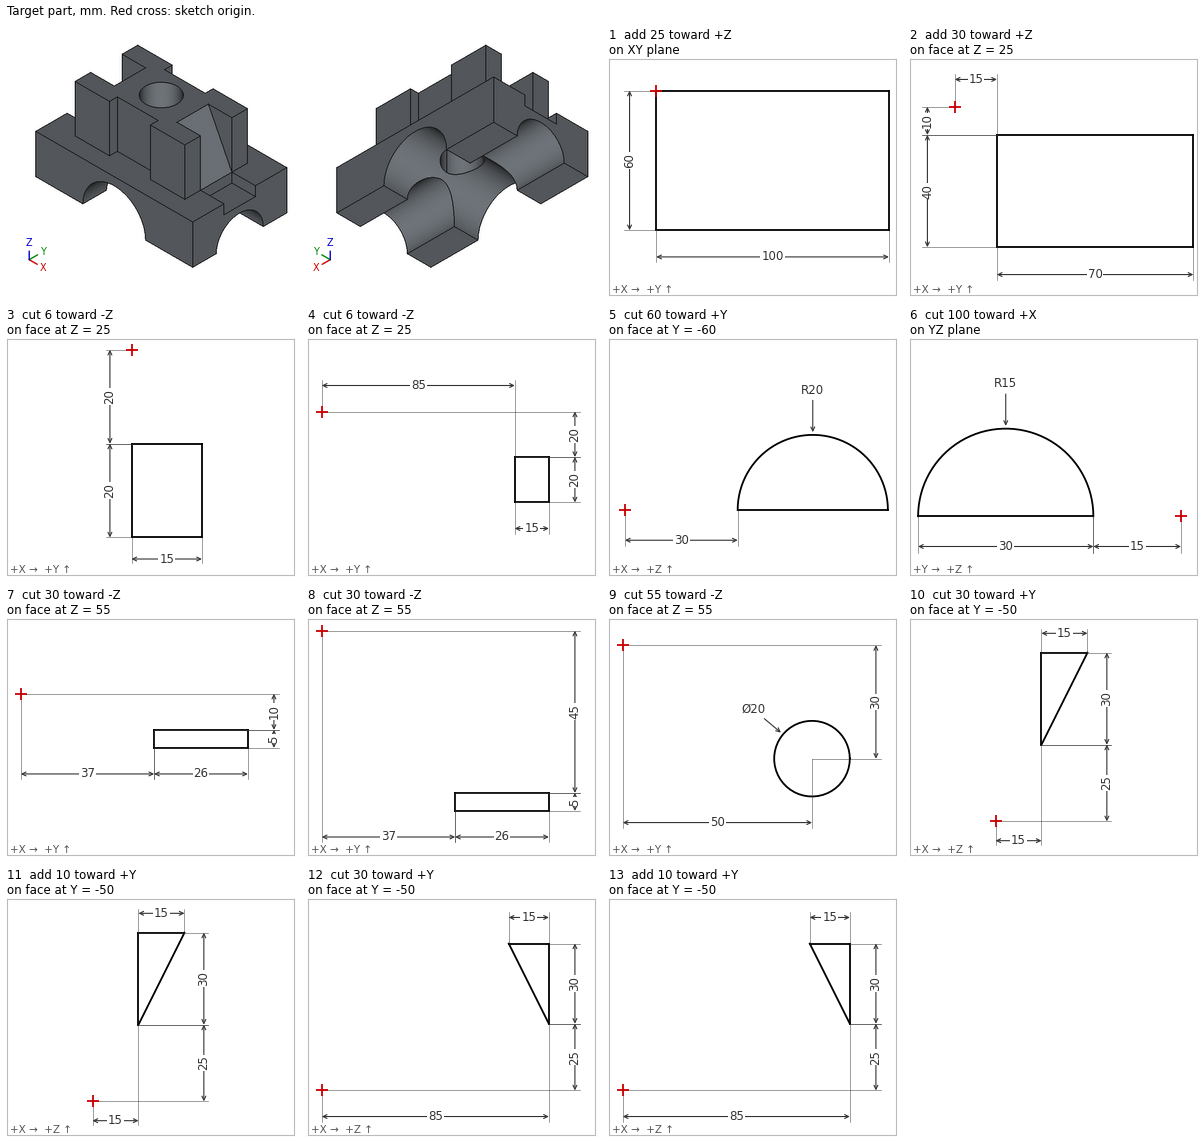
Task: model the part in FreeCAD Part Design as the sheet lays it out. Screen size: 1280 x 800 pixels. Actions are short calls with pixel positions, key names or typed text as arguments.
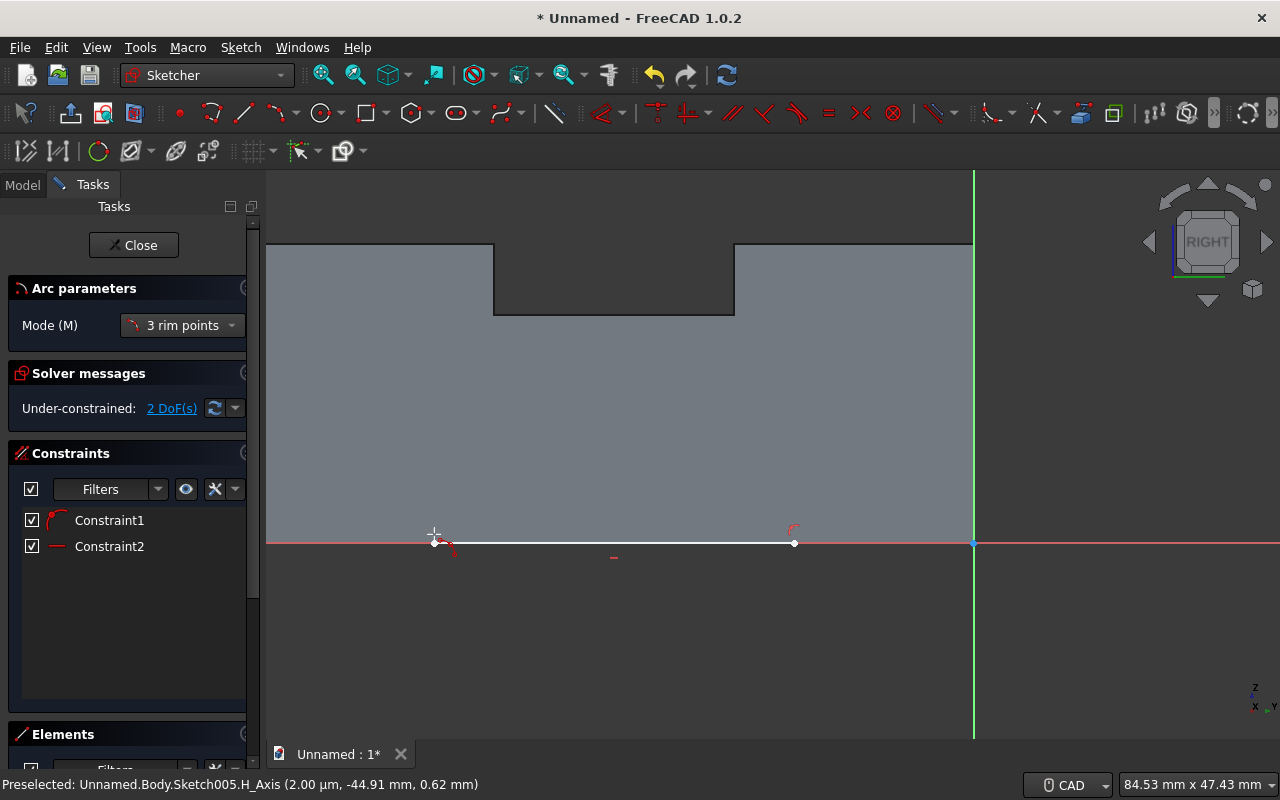
click(434, 534)
click(794, 543)
click(614, 363)
key(Escape)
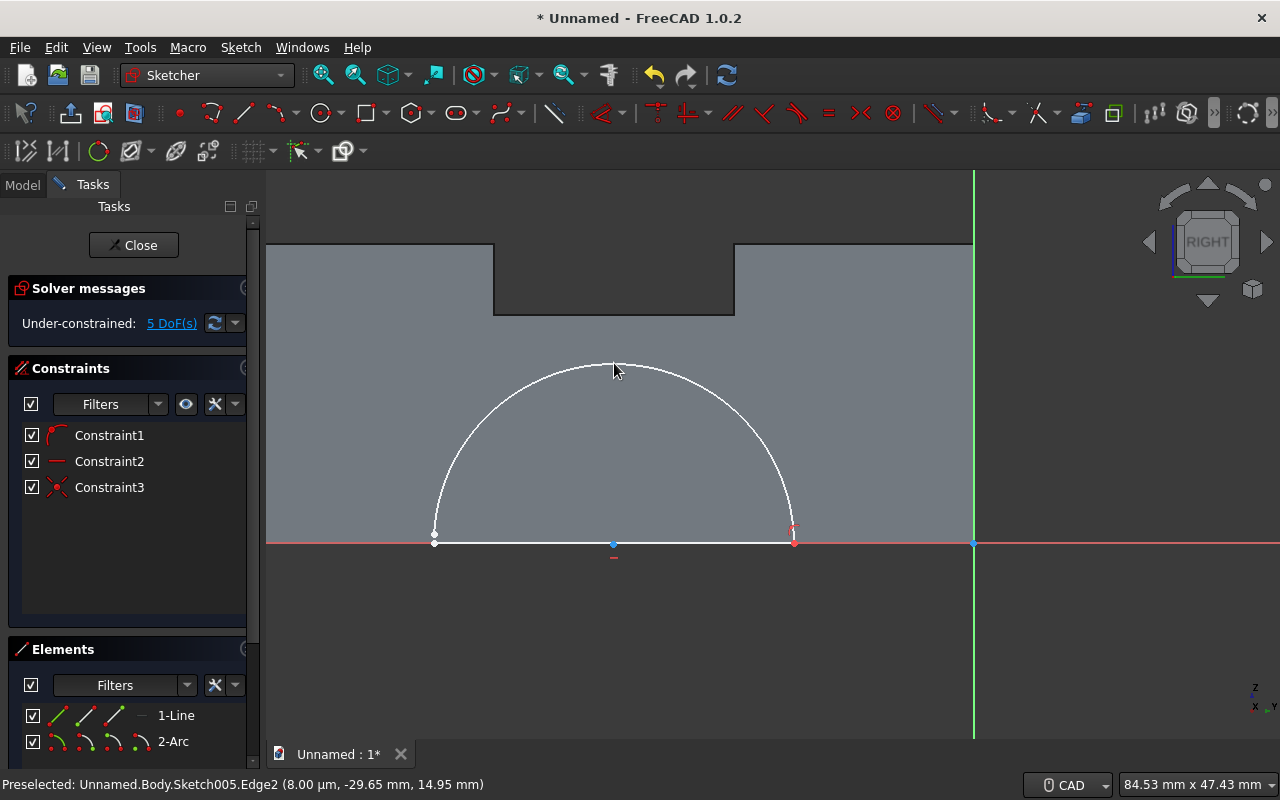
click(614, 544)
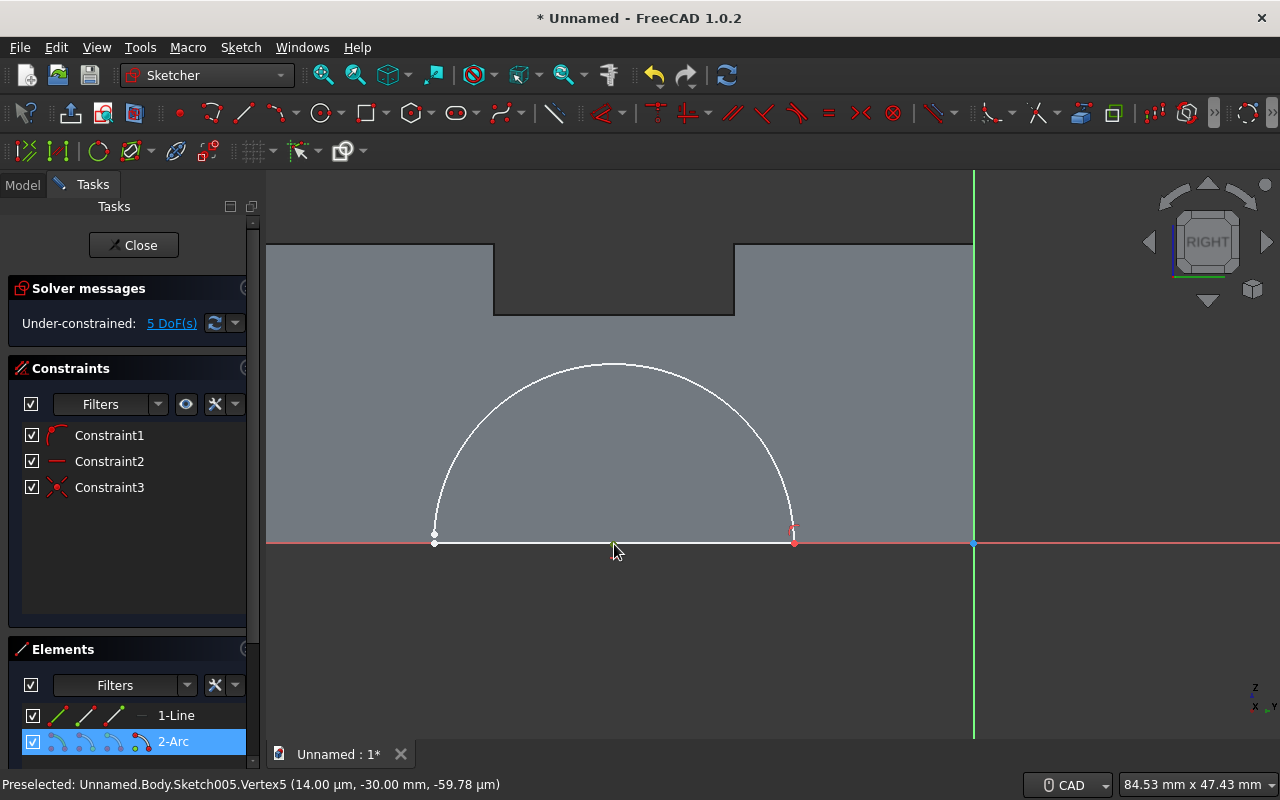
click(353, 543)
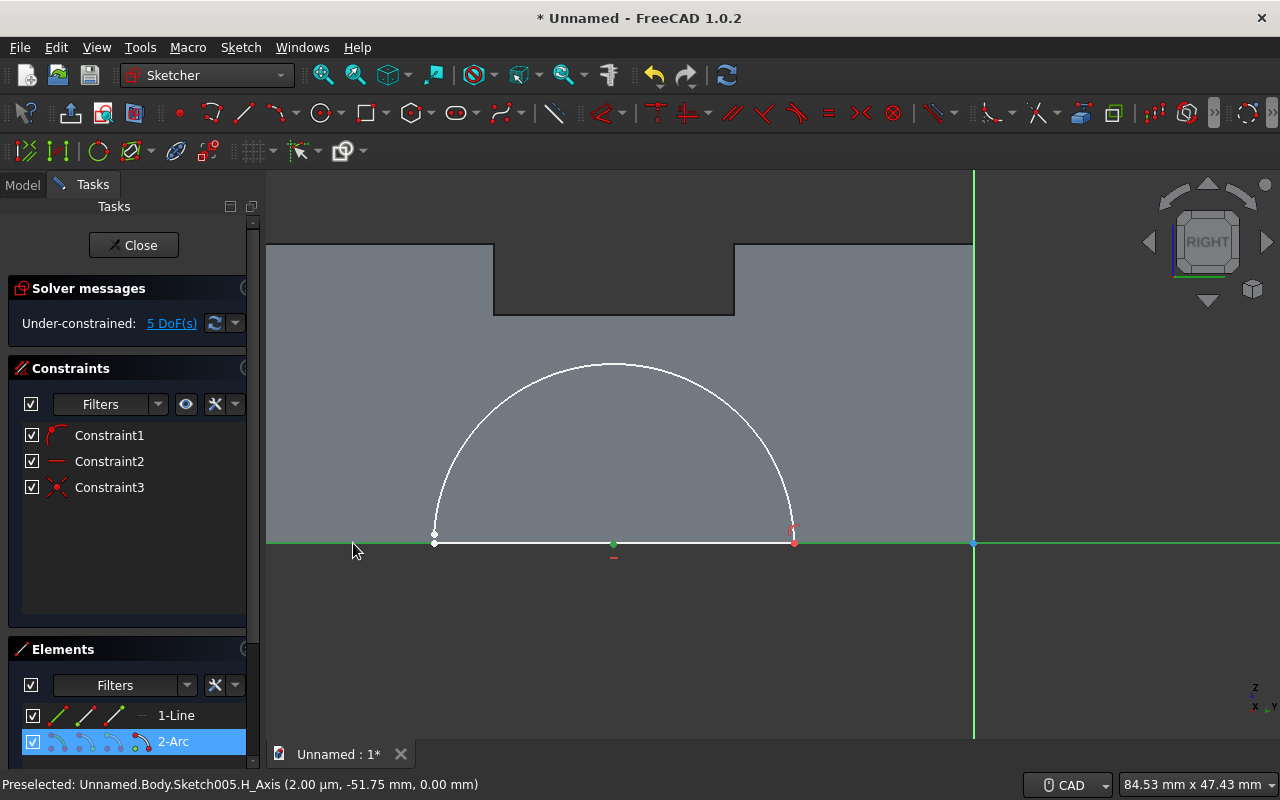
click(656, 114)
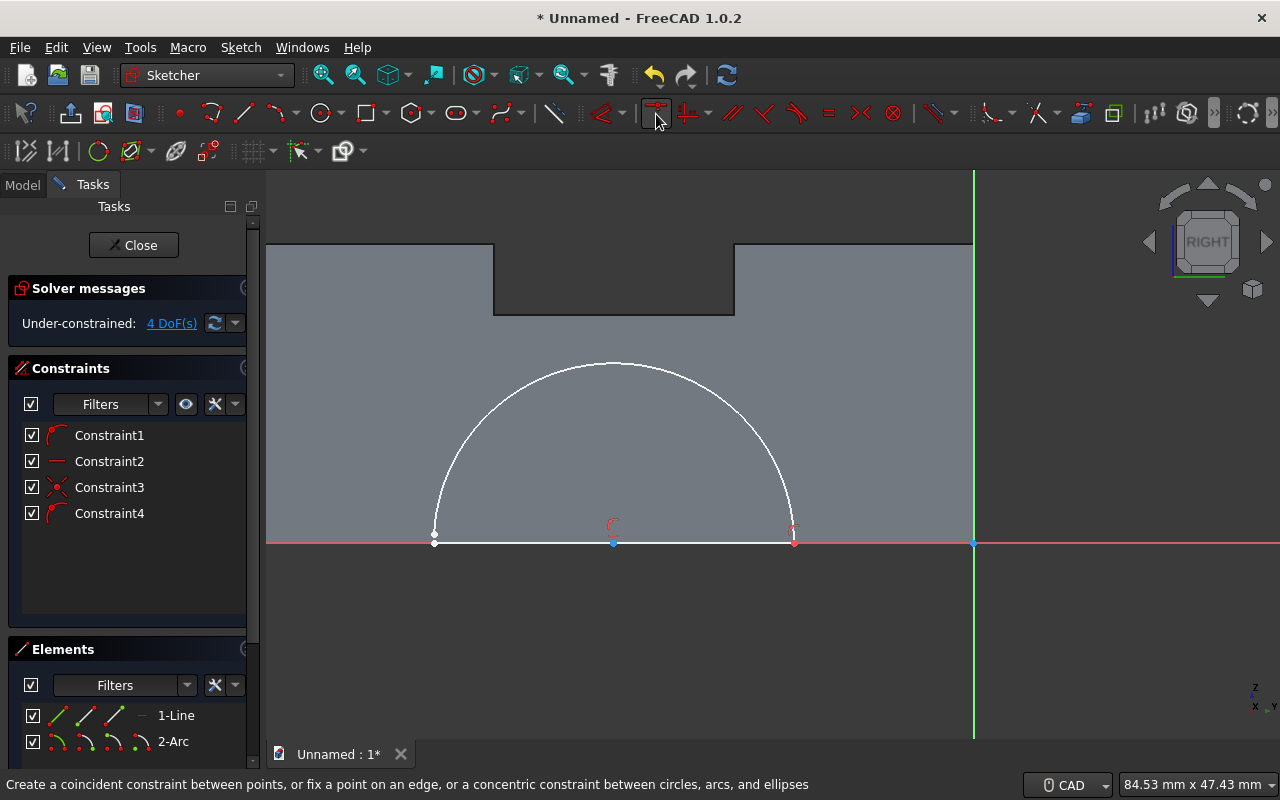
key(d)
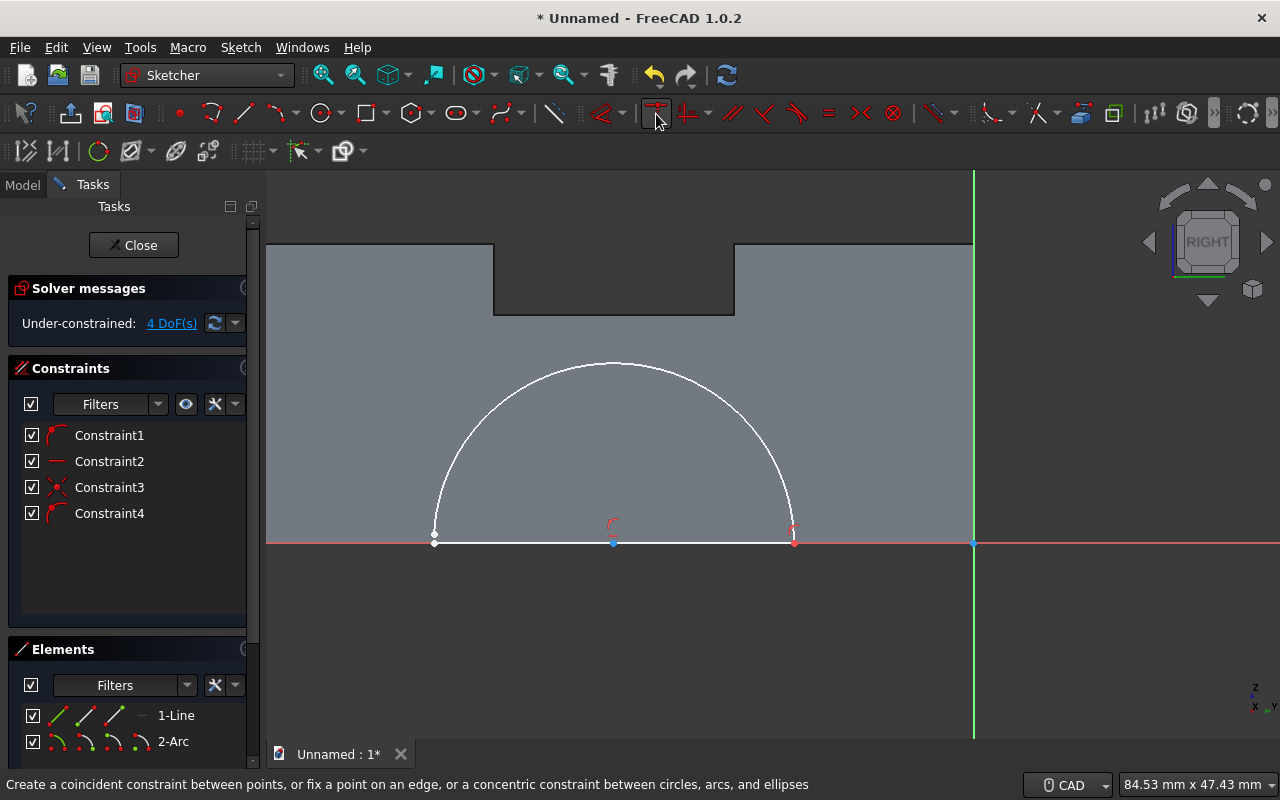
click(722, 399)
click(741, 373)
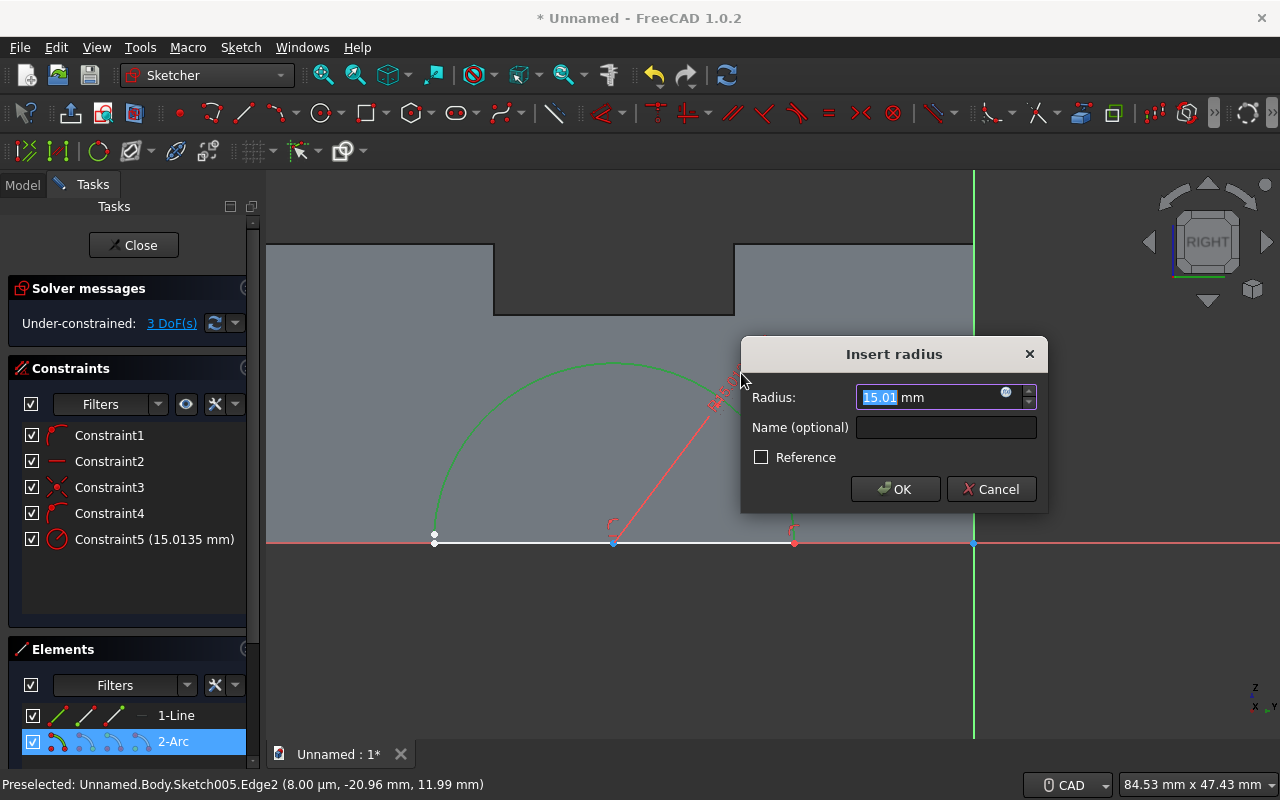
text(15)
key(Return)
key(Escape)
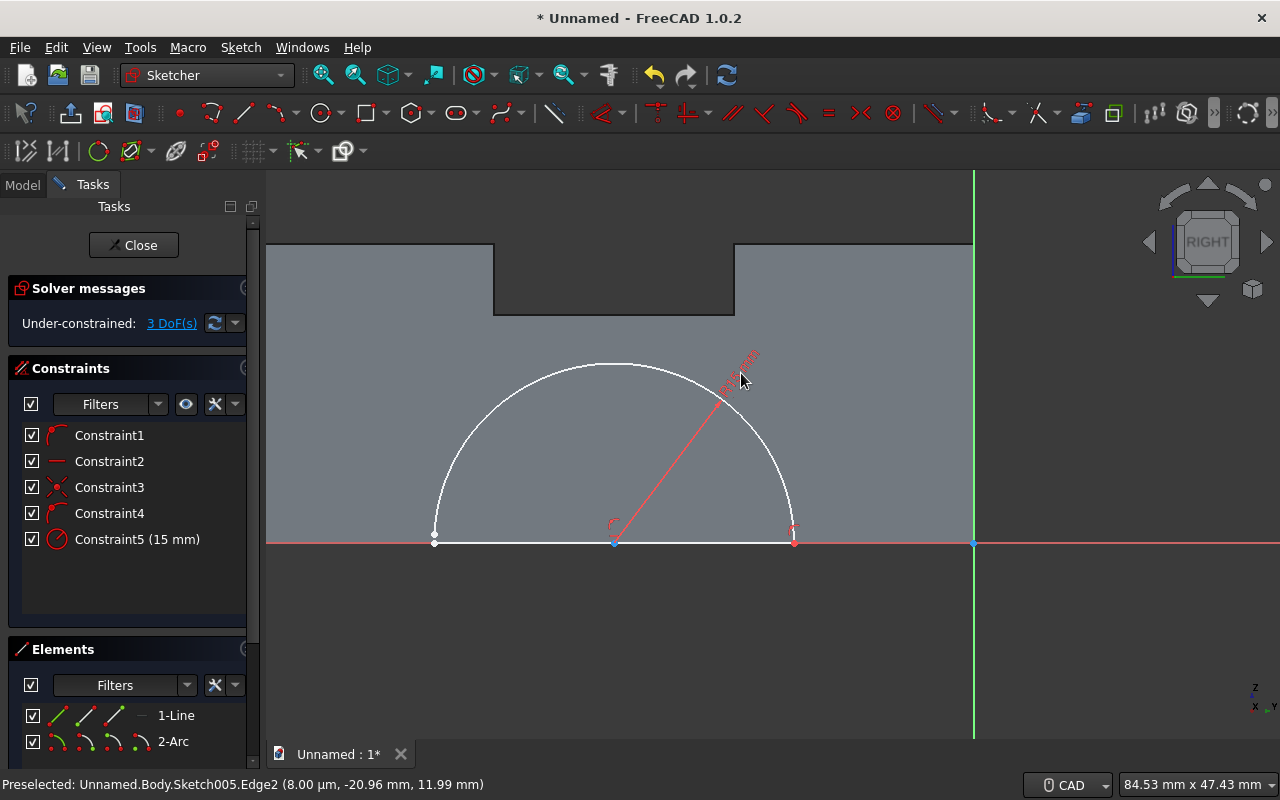
click(434, 535)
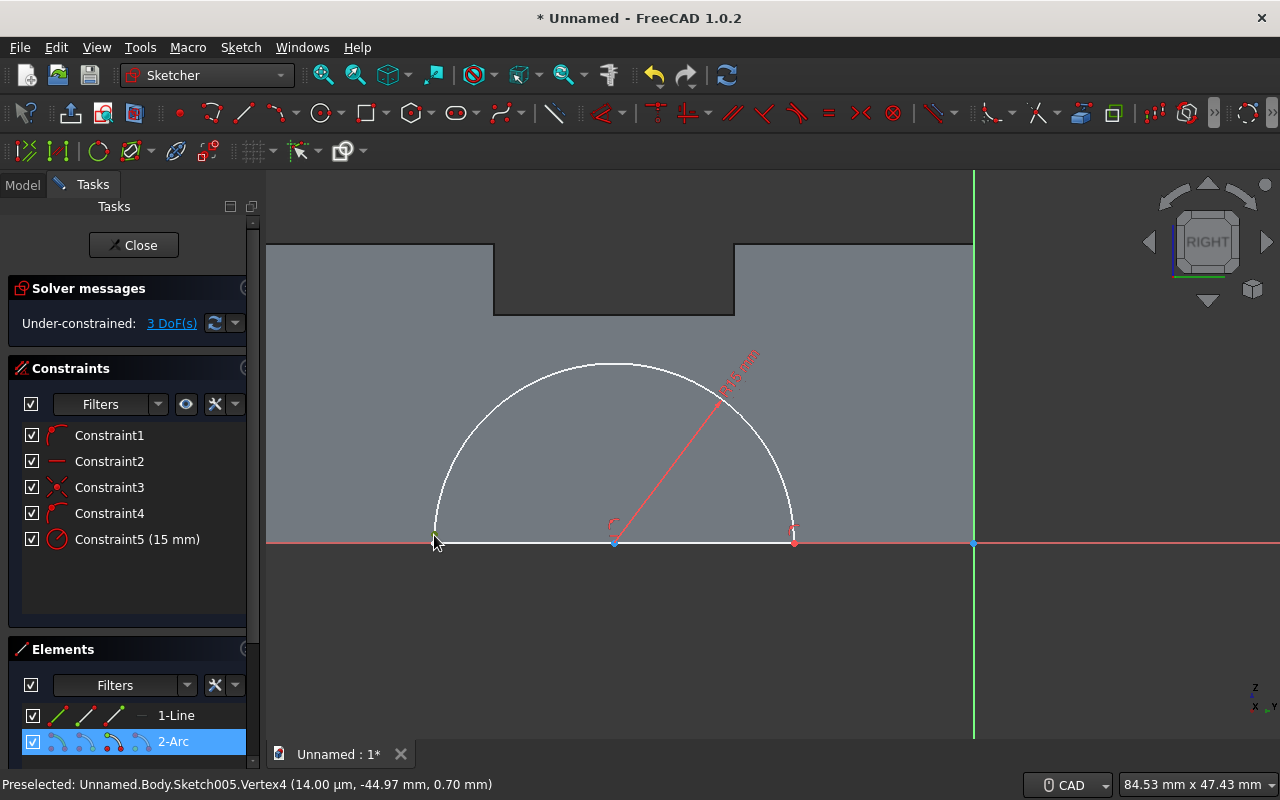
click(353, 543)